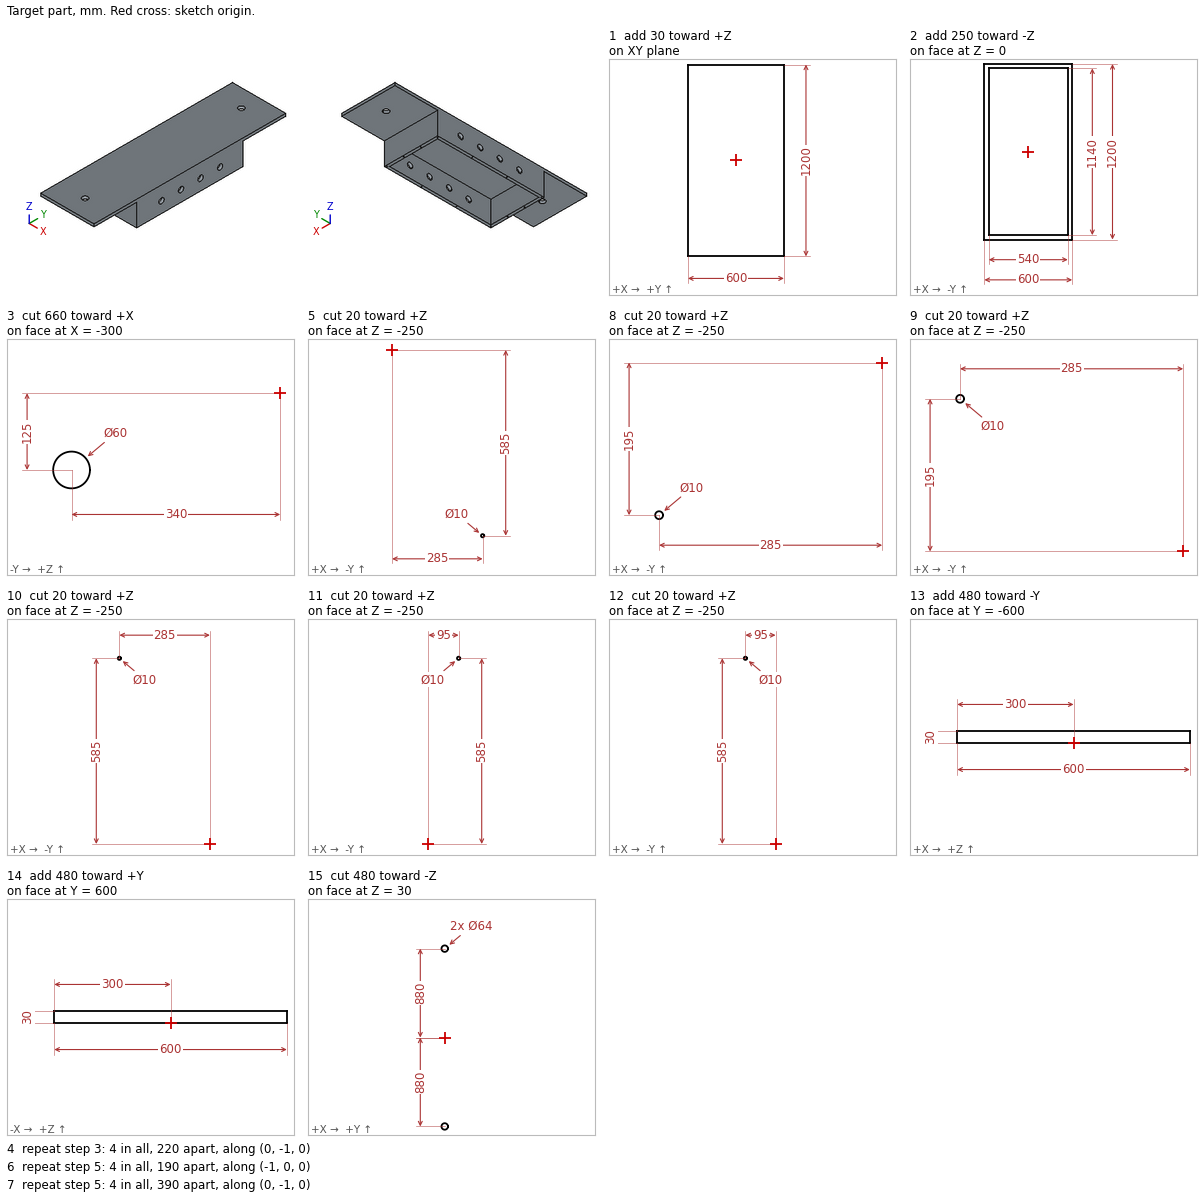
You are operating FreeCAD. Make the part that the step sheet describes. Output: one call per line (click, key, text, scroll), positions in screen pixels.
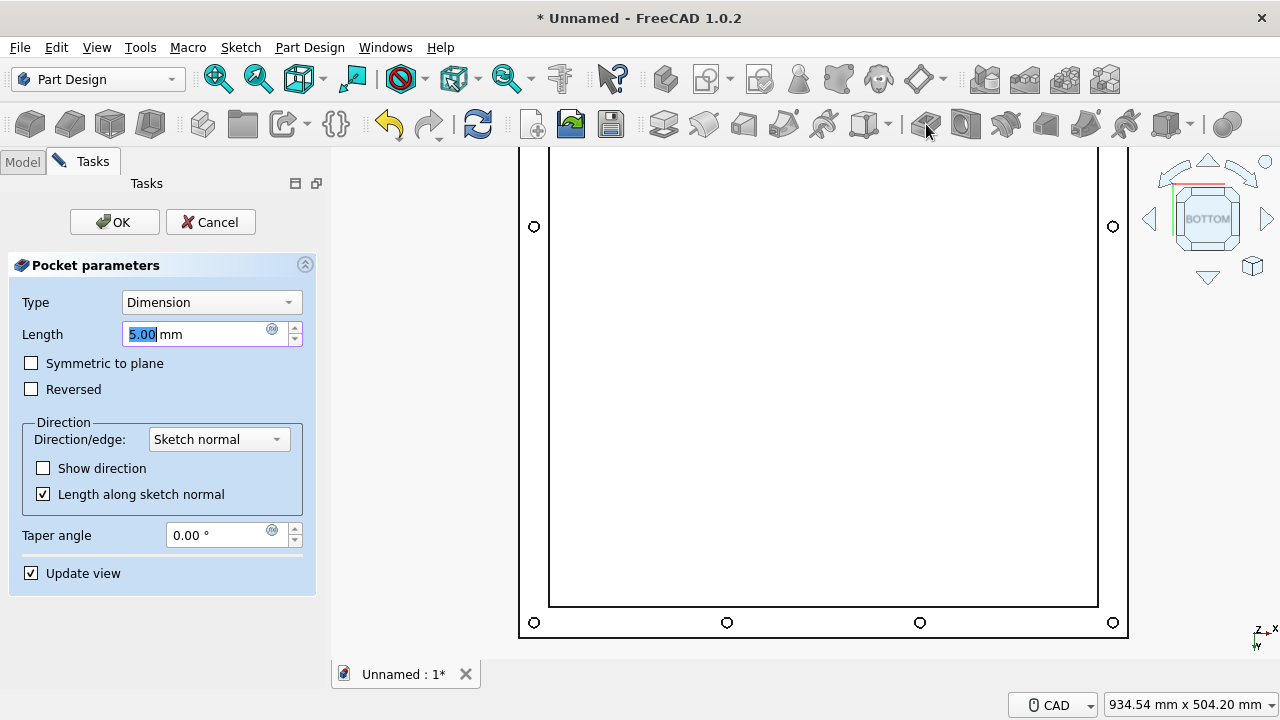
text(20)
key(Tab)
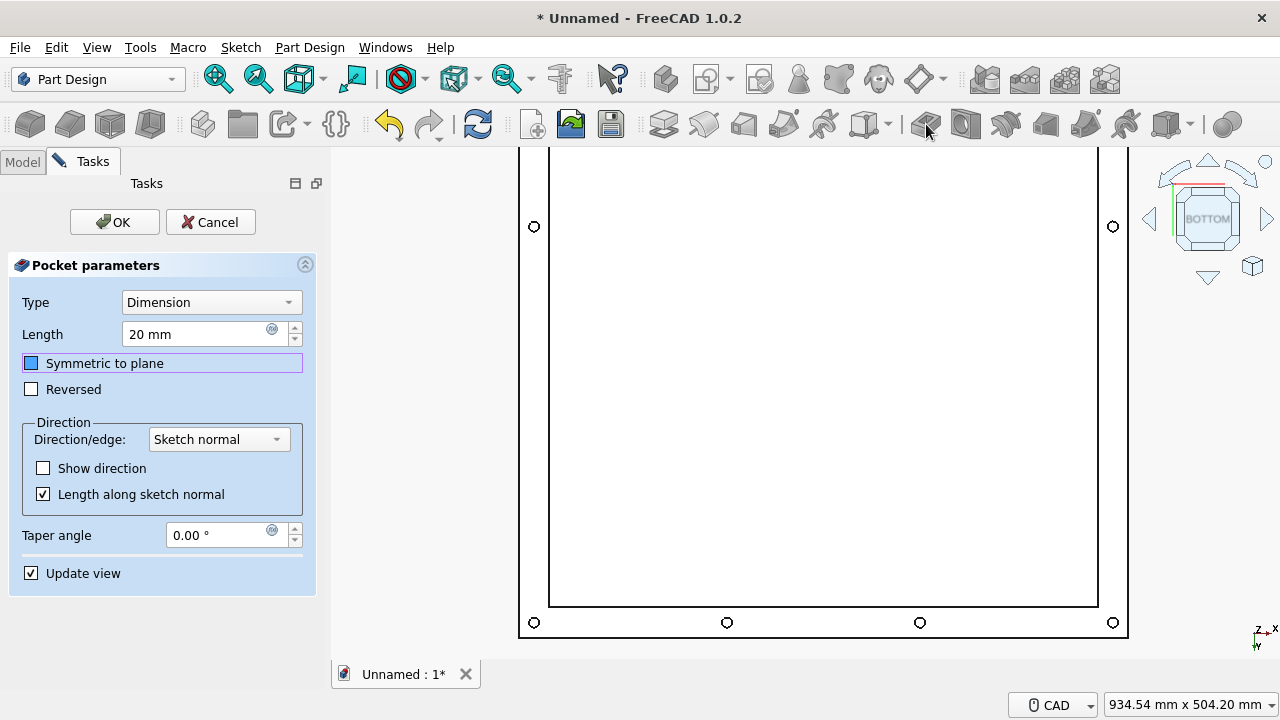
click(115, 222)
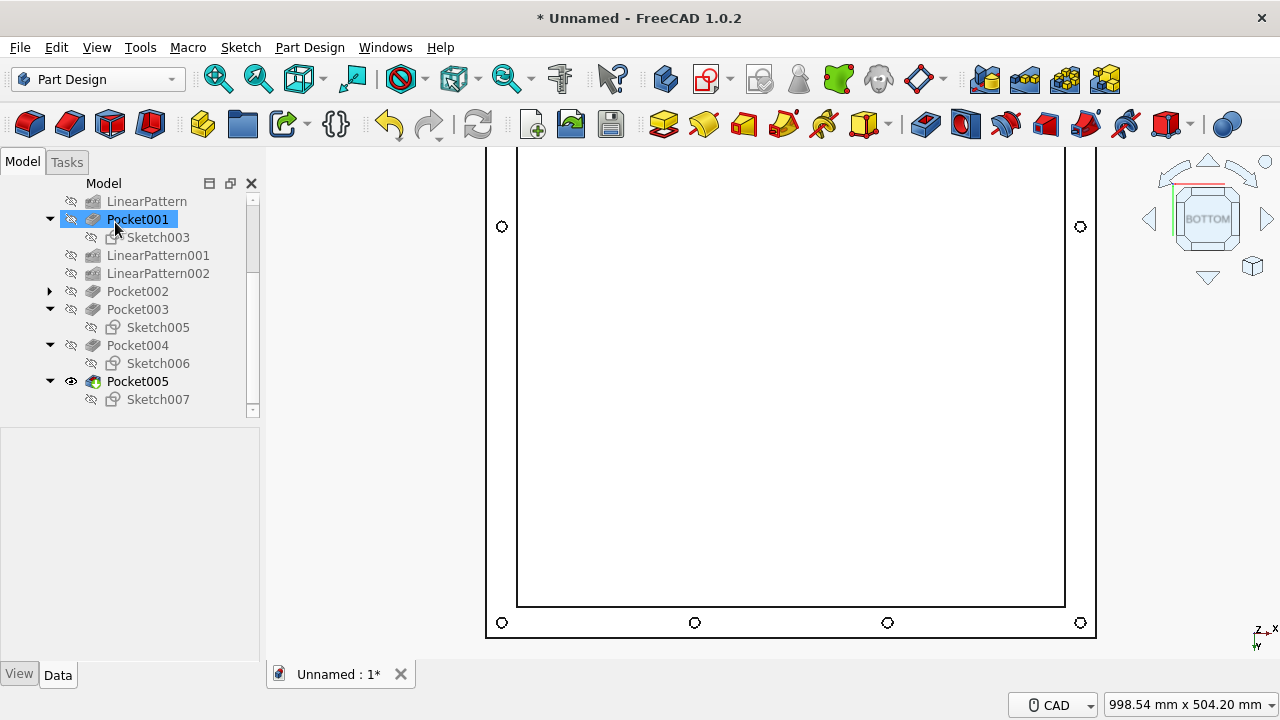
click(220, 80)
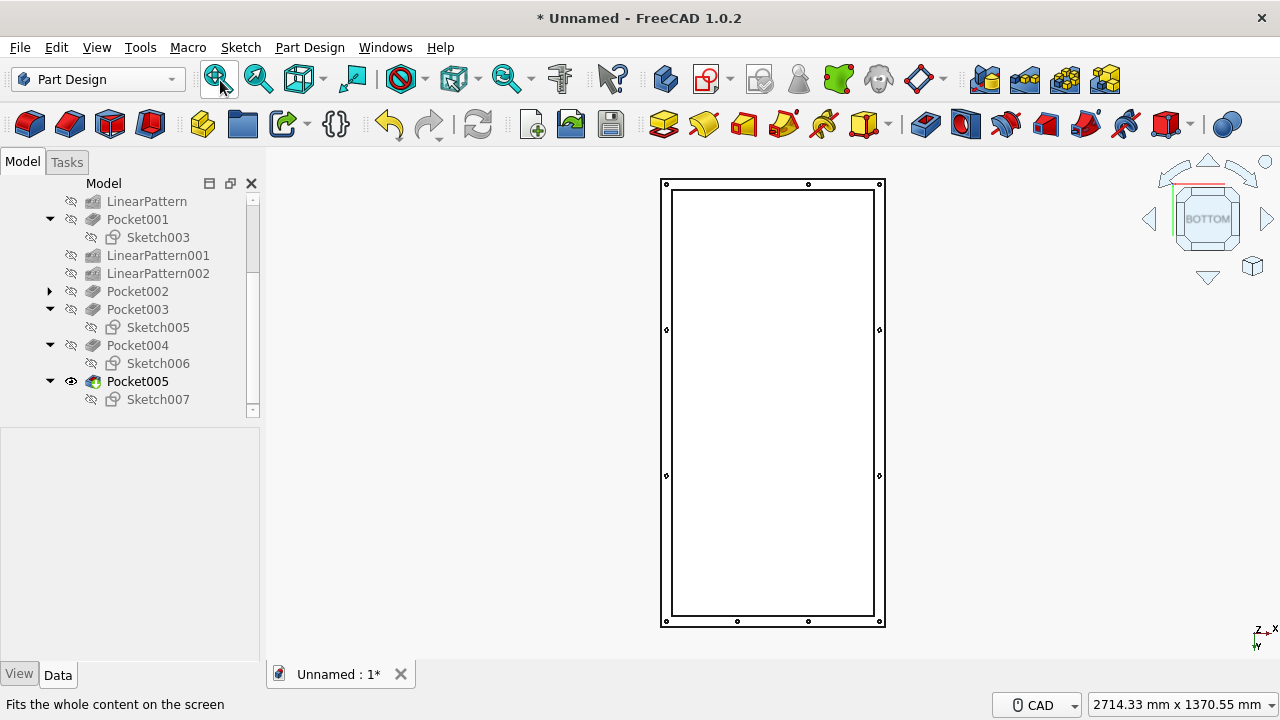
scroll(762, 621, up, 5)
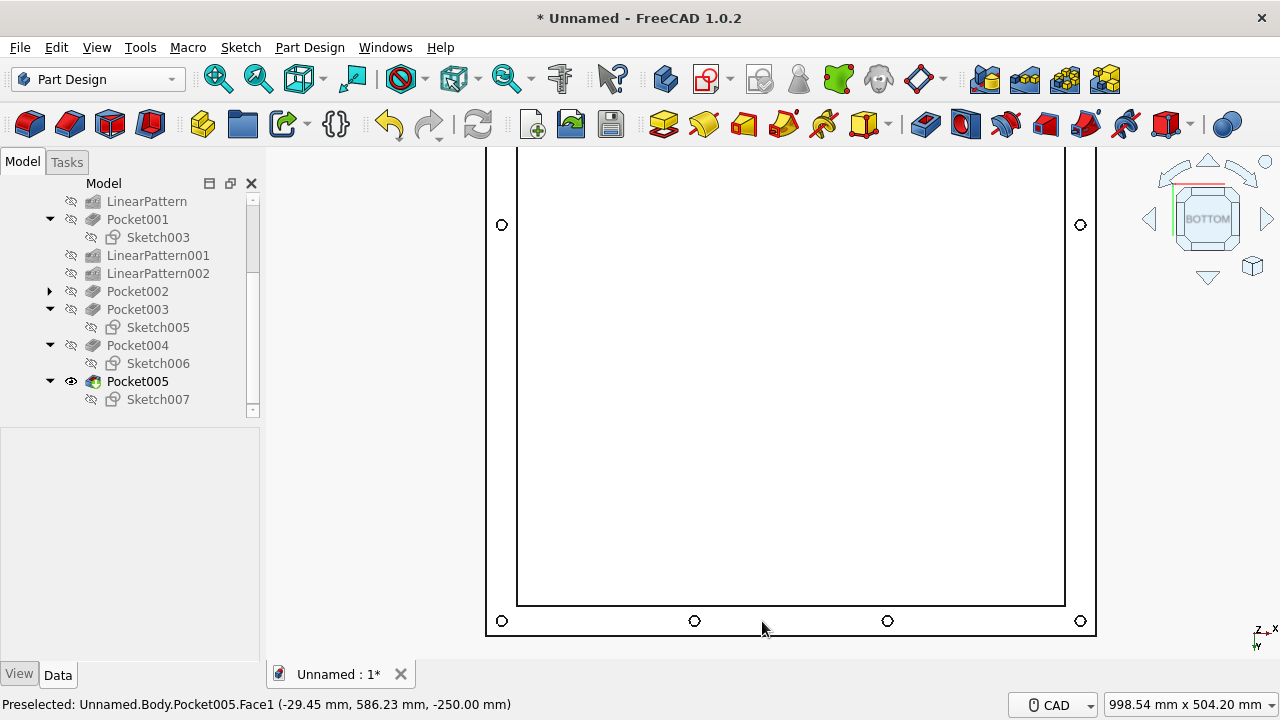
click(760, 621)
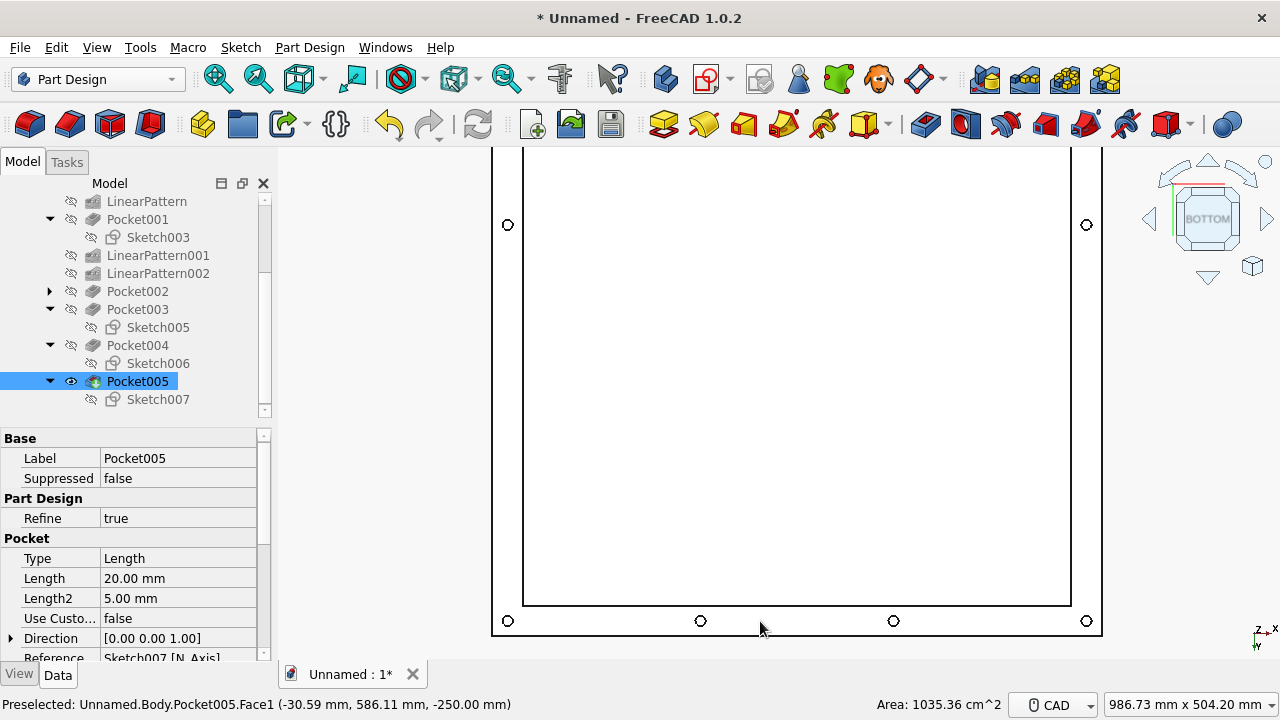
click(706, 80)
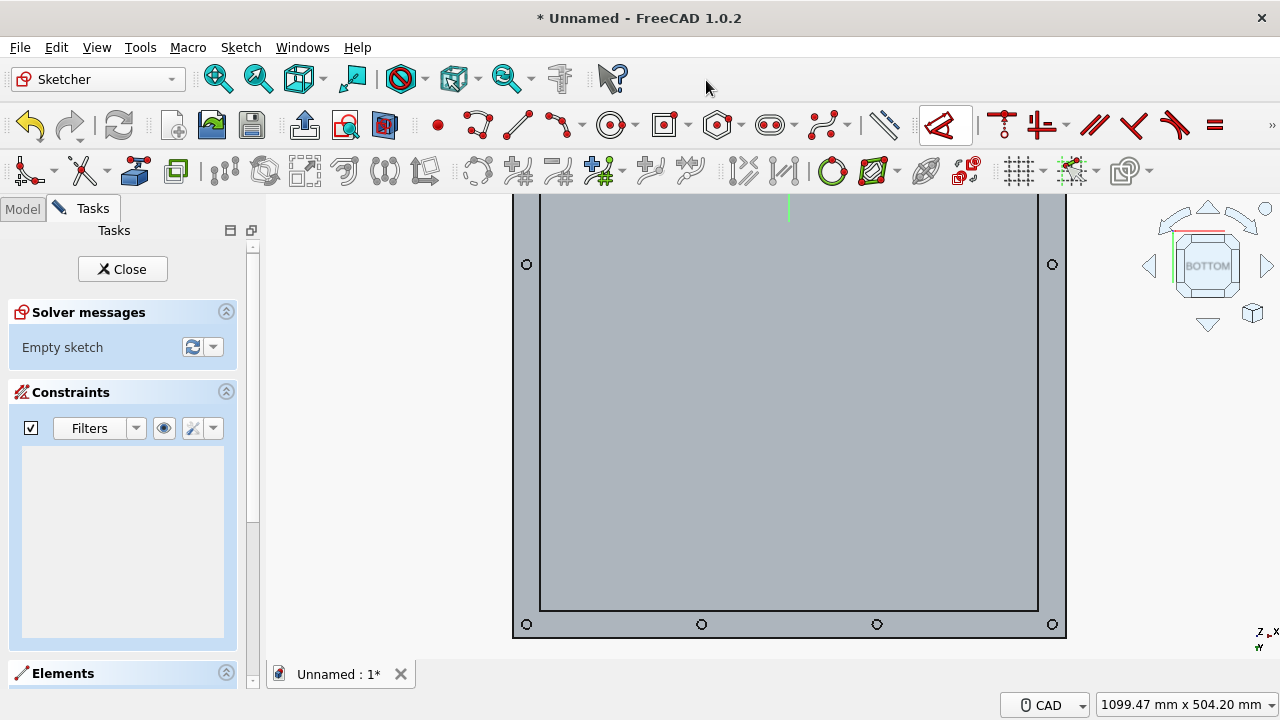
scroll(704, 426, down, 5)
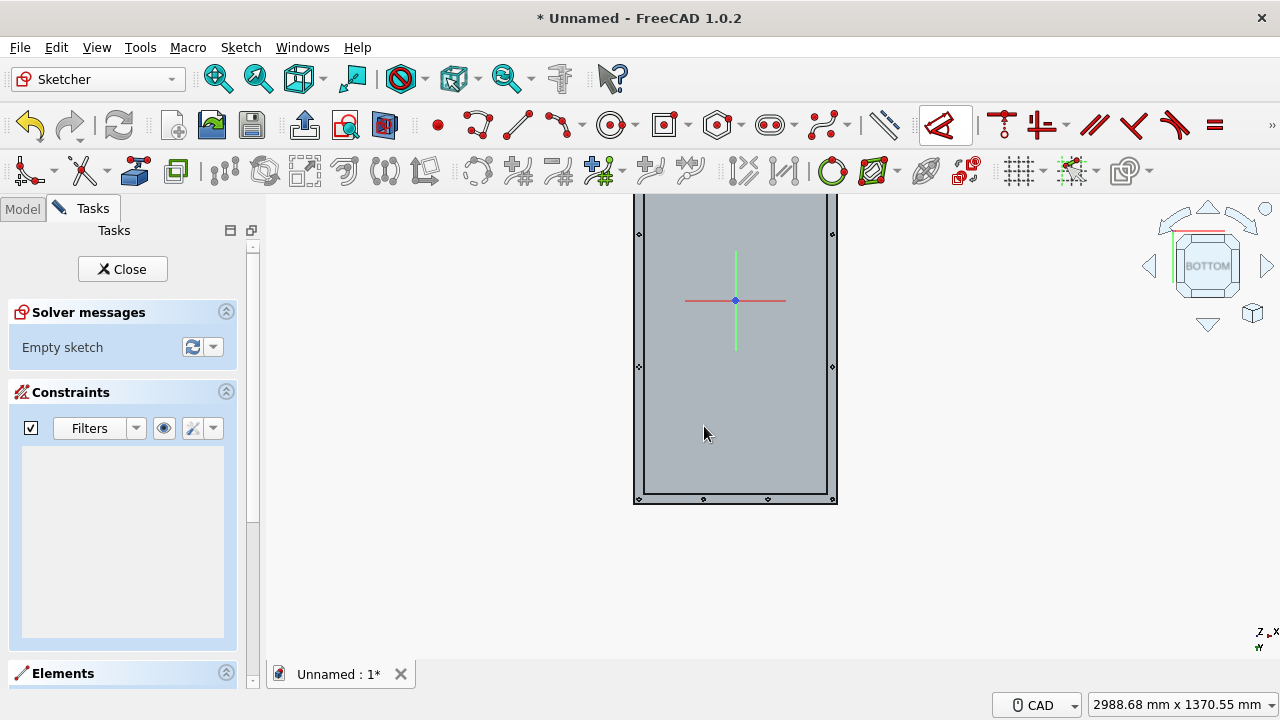
scroll(704, 426, down, 5)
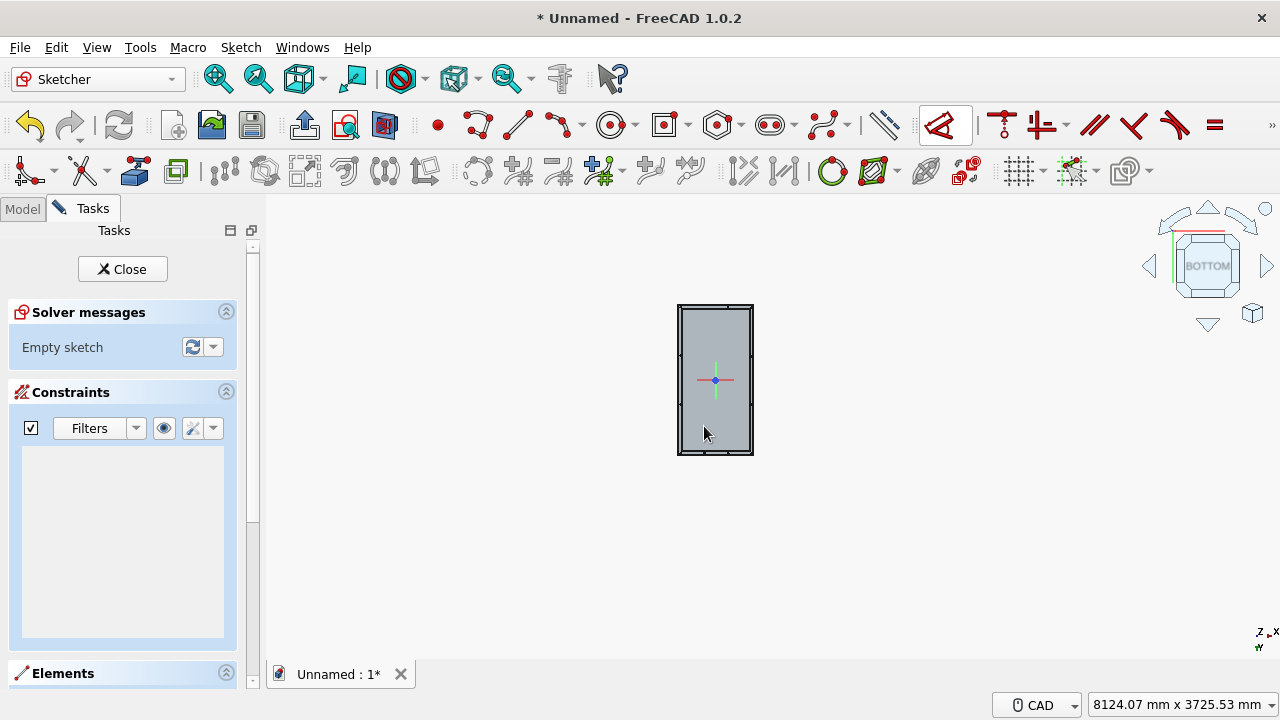
scroll(704, 301, up, 15)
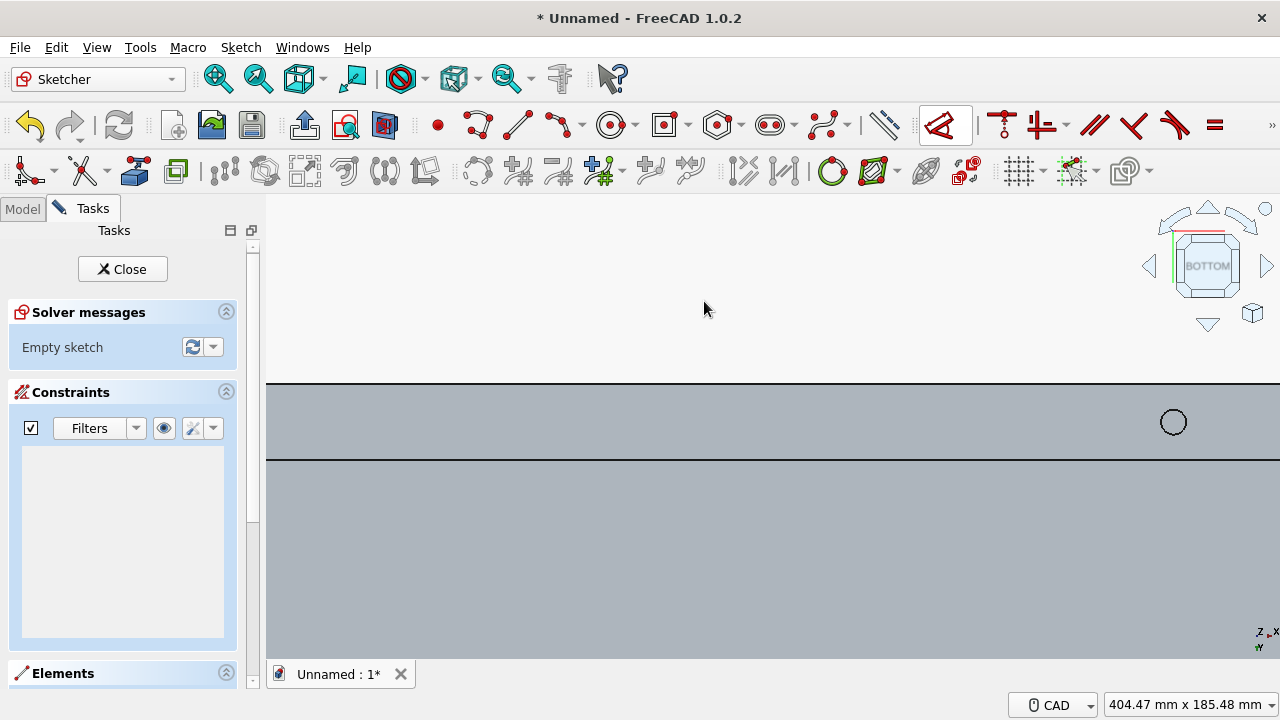
scroll(697, 422, up, 12)